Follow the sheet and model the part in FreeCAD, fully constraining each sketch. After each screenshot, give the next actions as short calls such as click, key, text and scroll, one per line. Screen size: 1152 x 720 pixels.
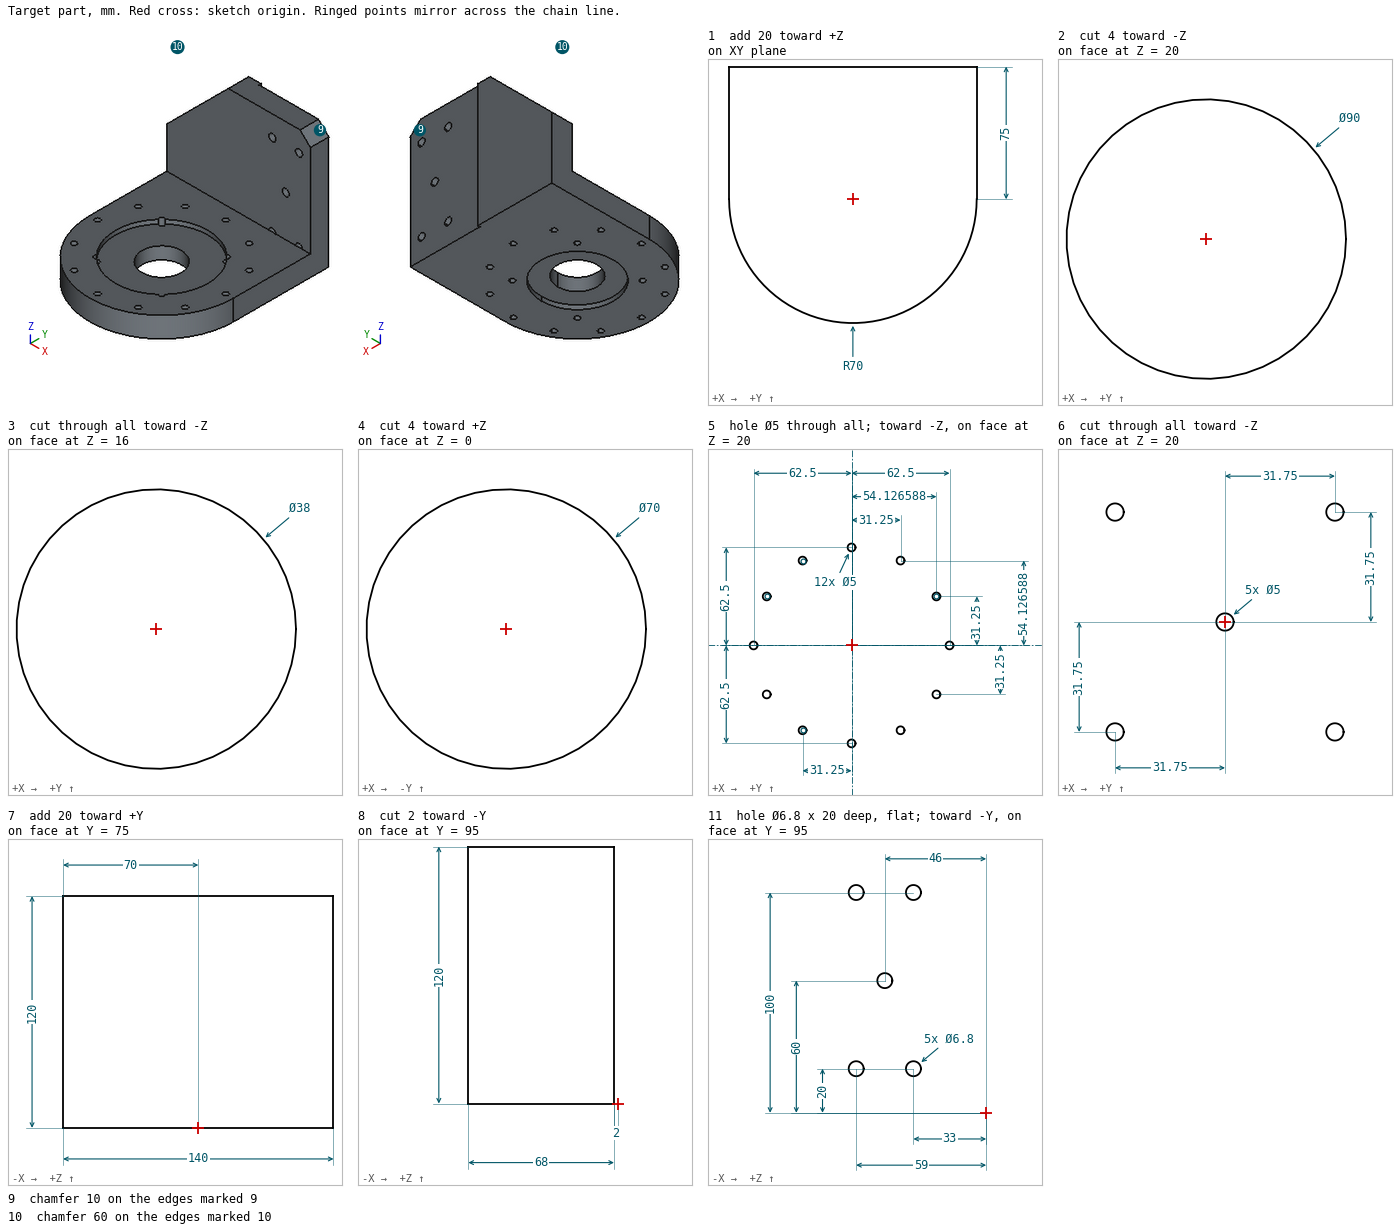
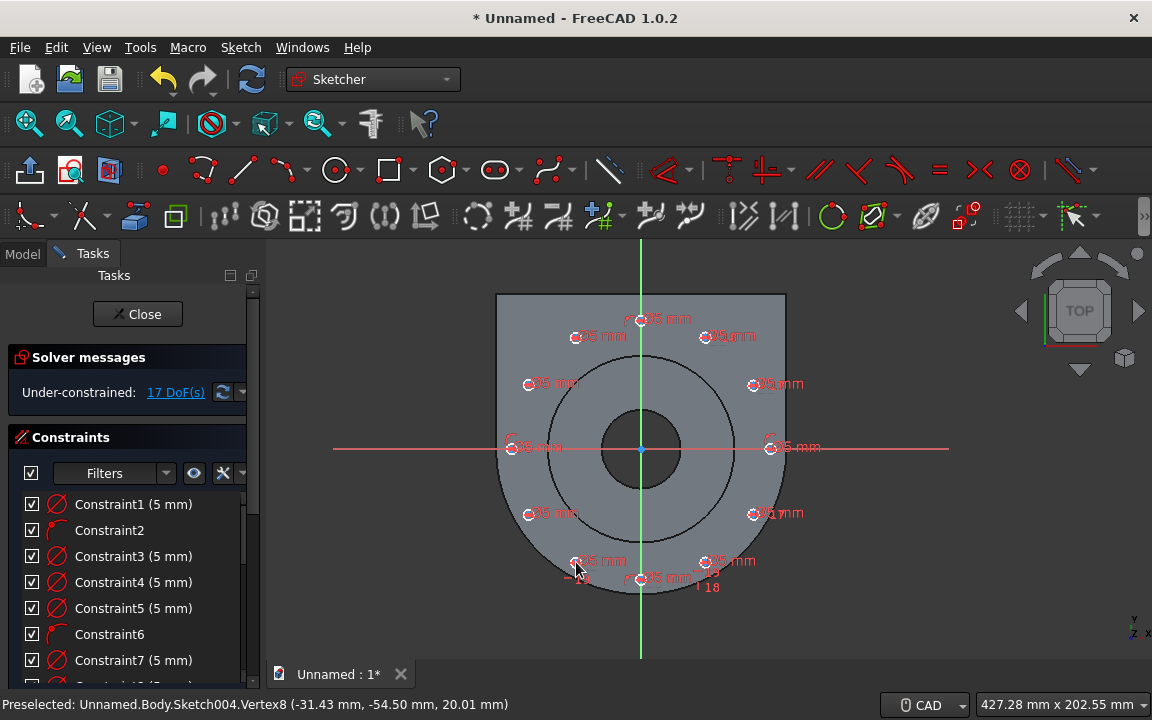
click(754, 515)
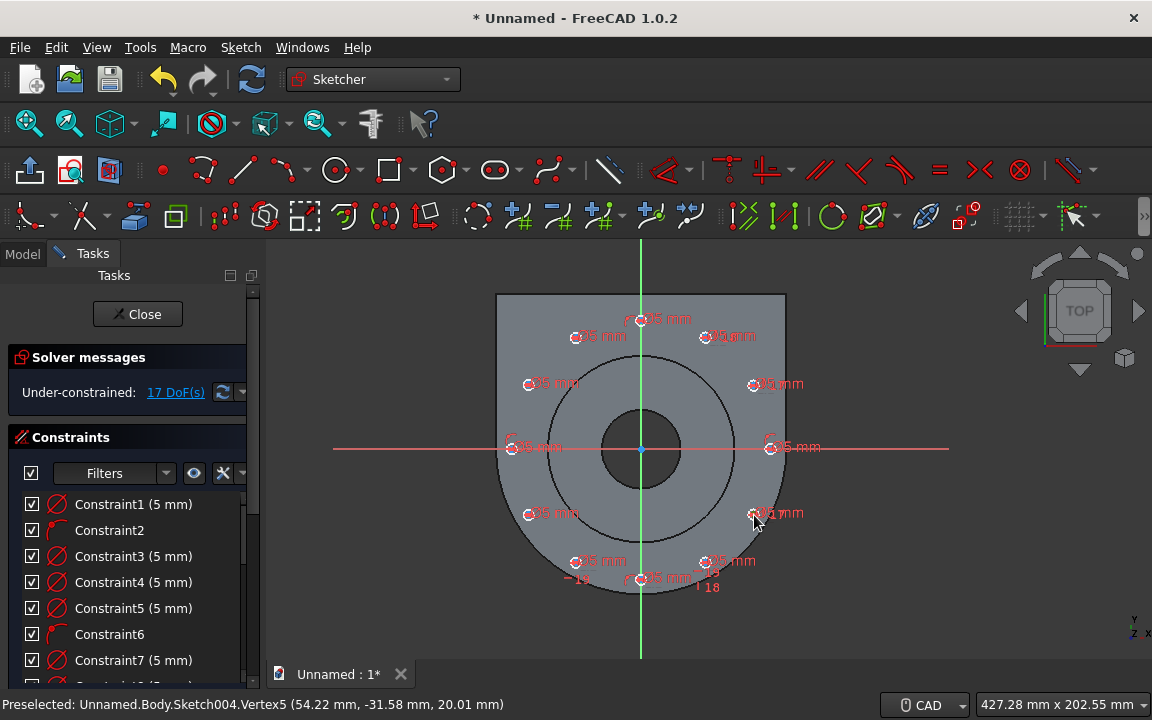
click(529, 515)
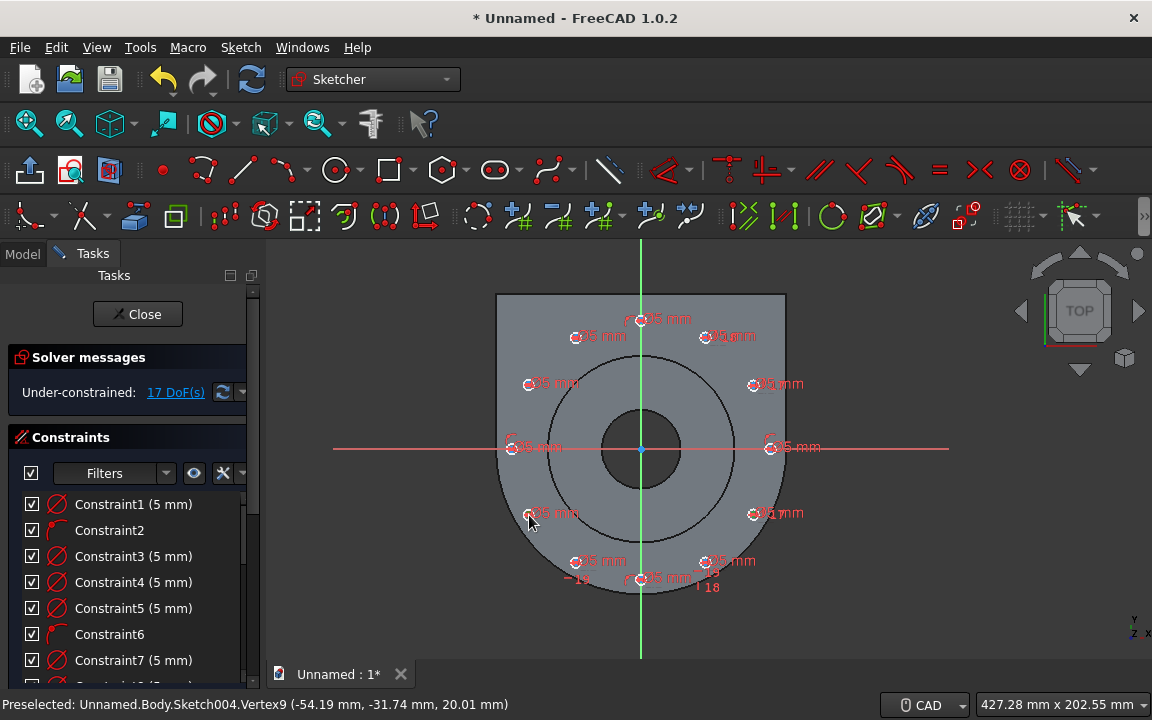
key(h)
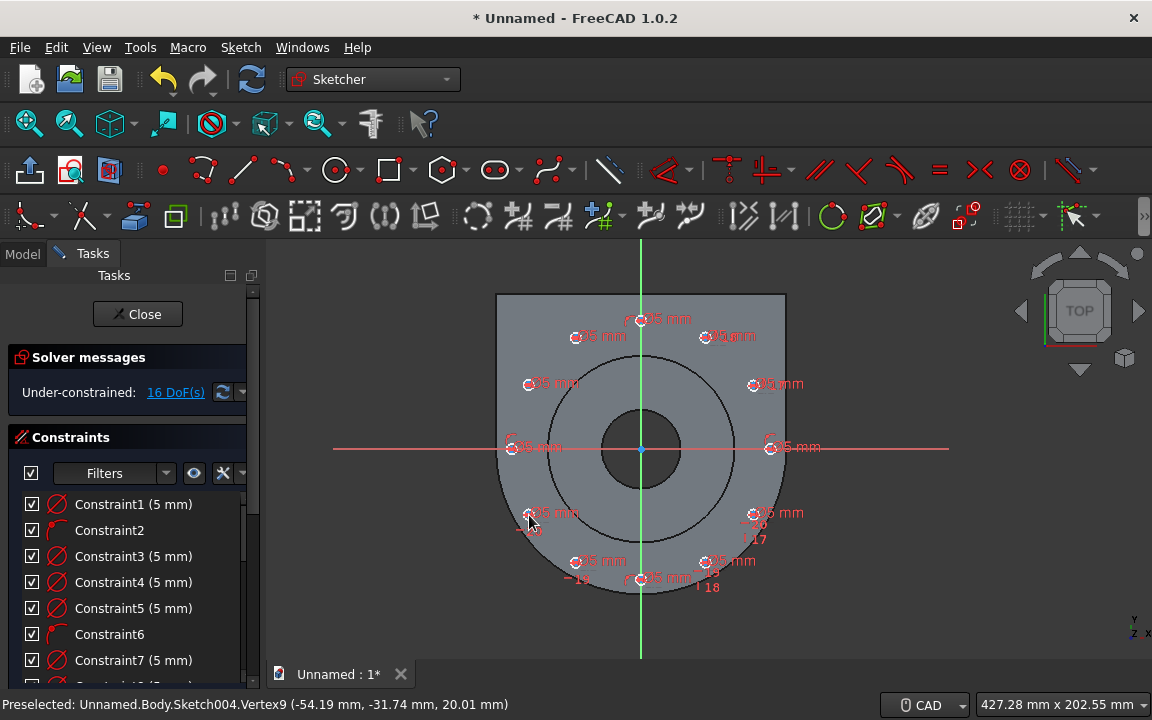
click(529, 515)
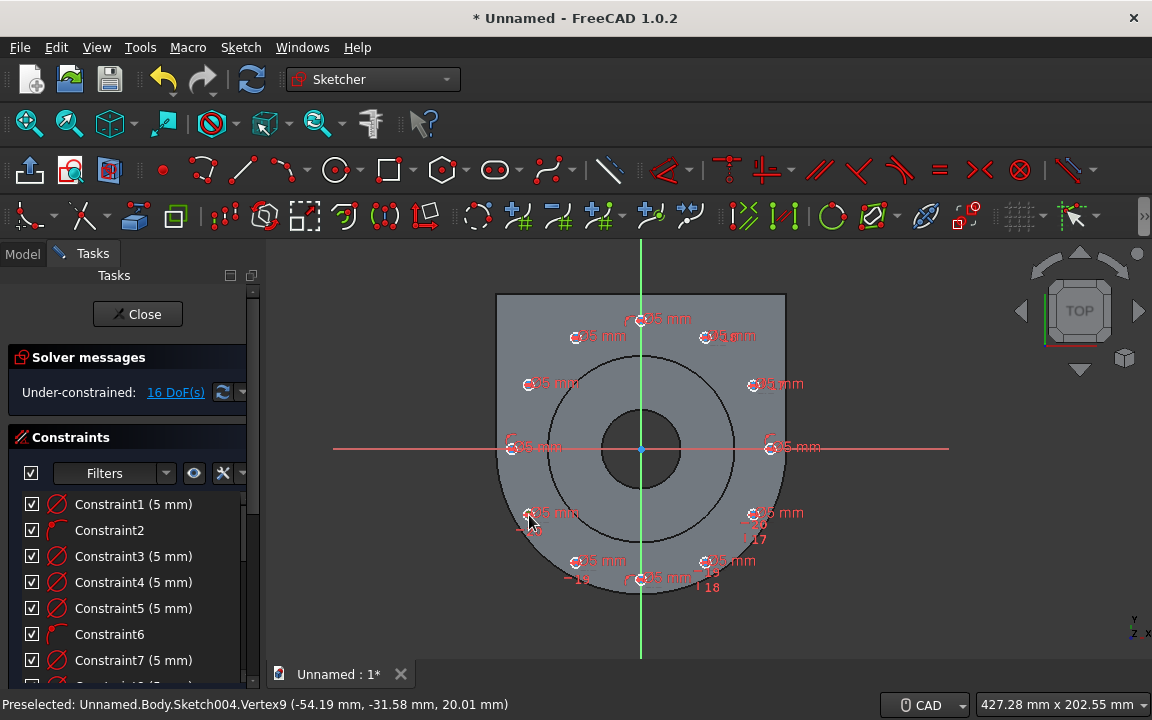
click(529, 385)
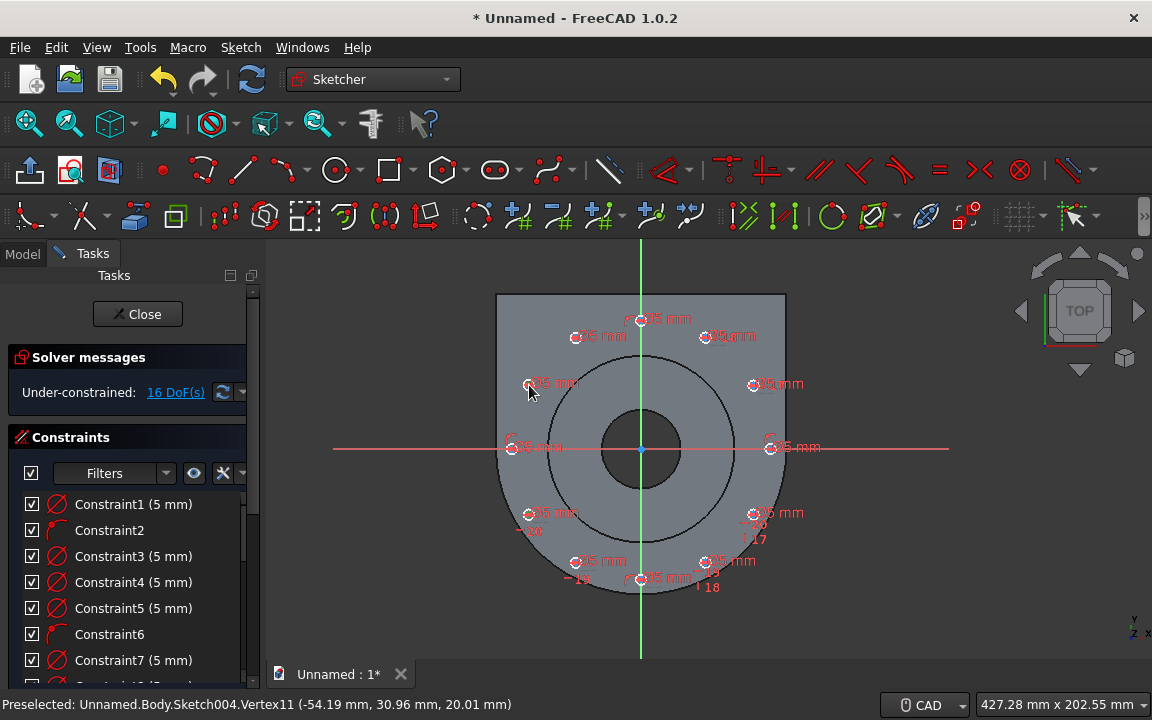
key(v)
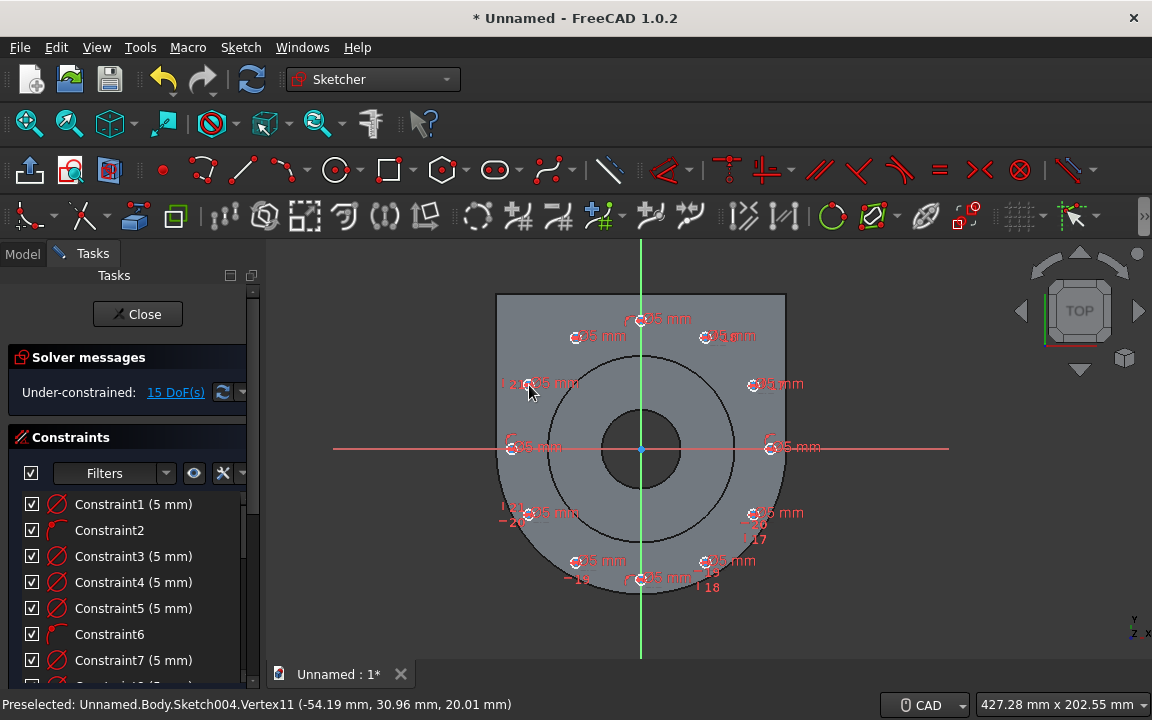
click(706, 338)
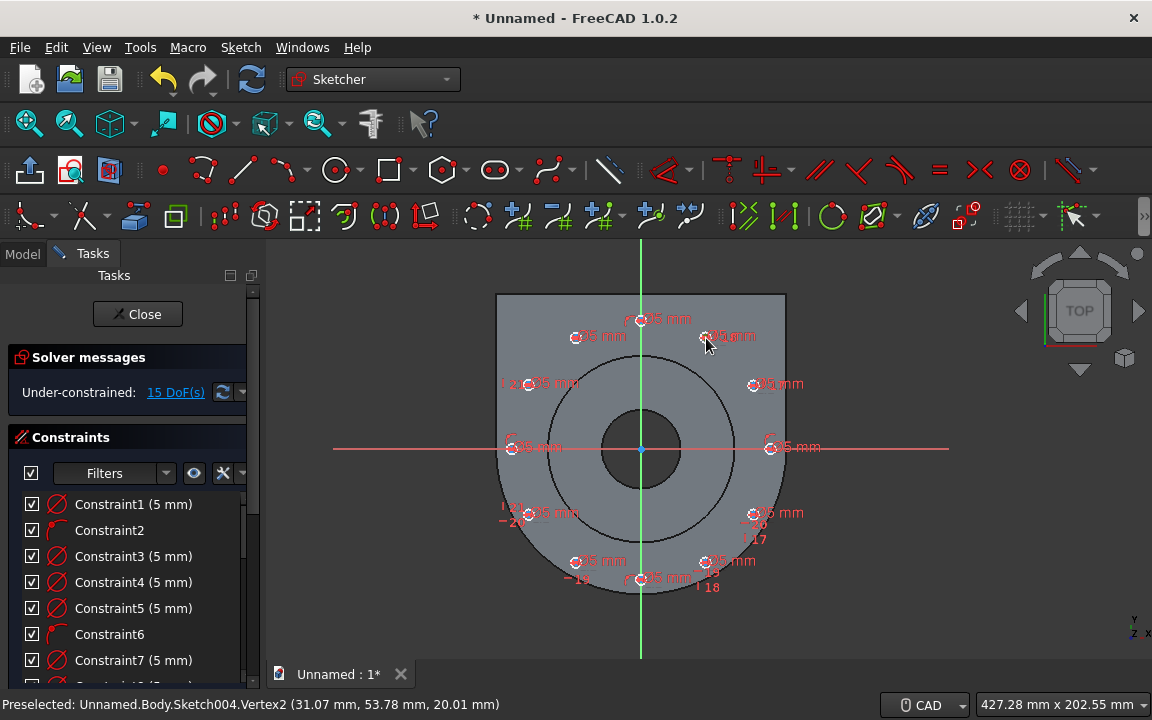
click(576, 338)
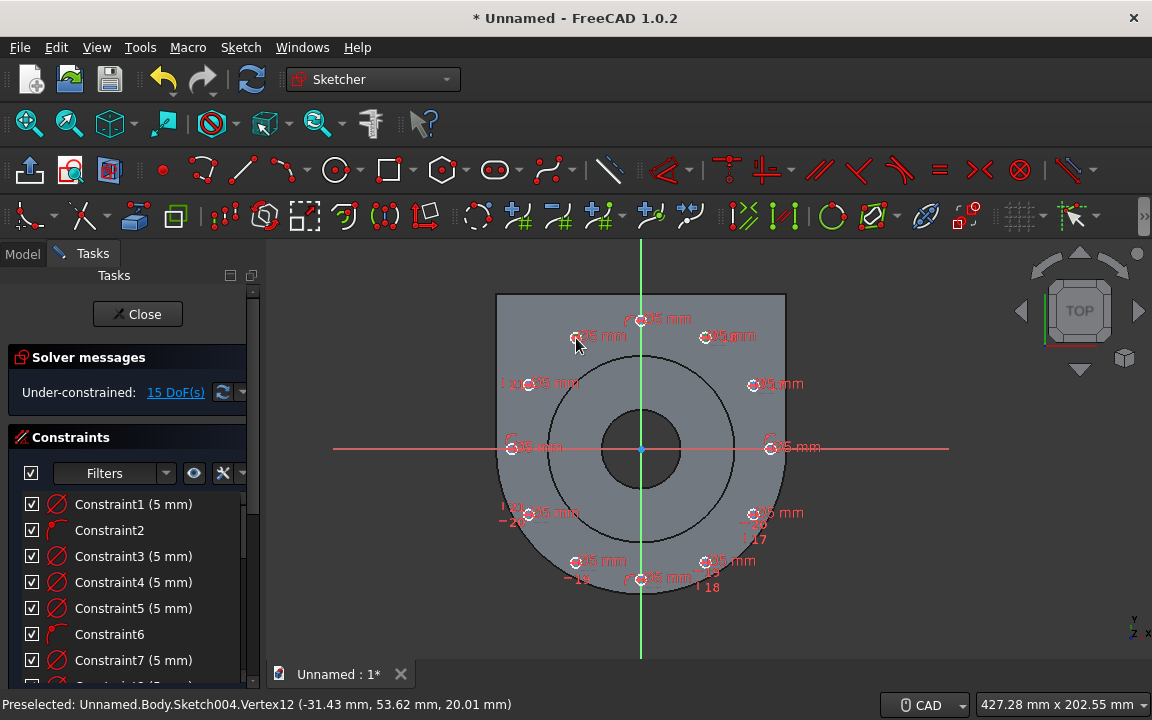
key(h)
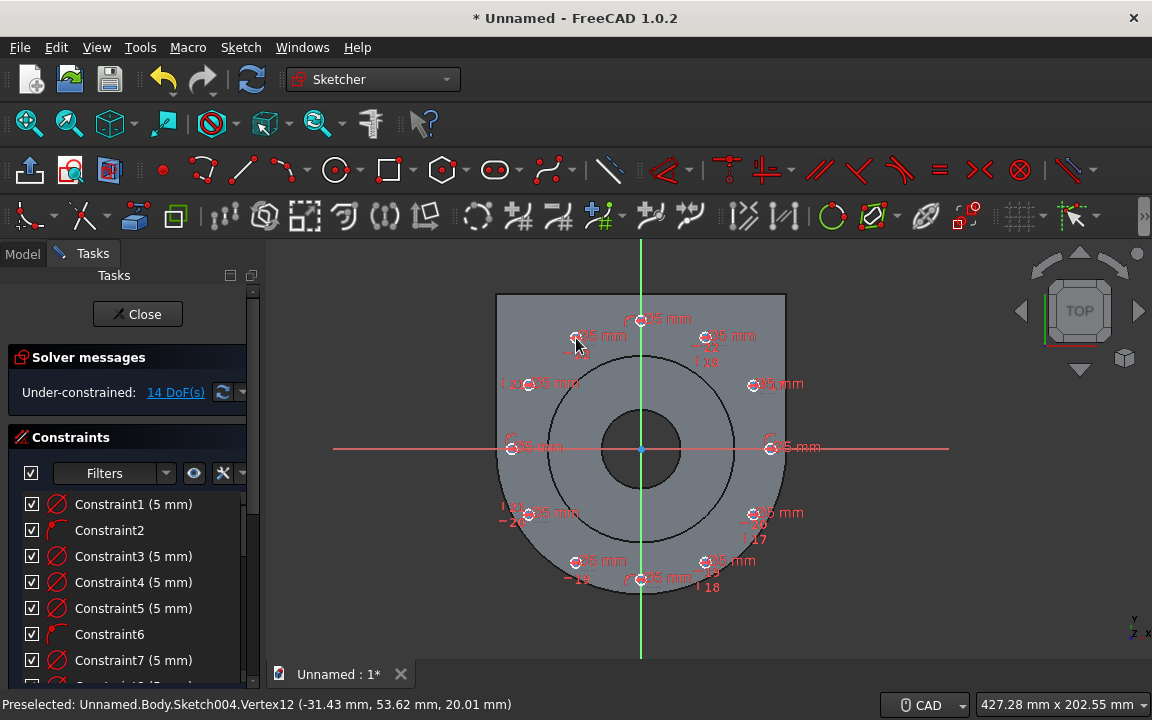
click(754, 386)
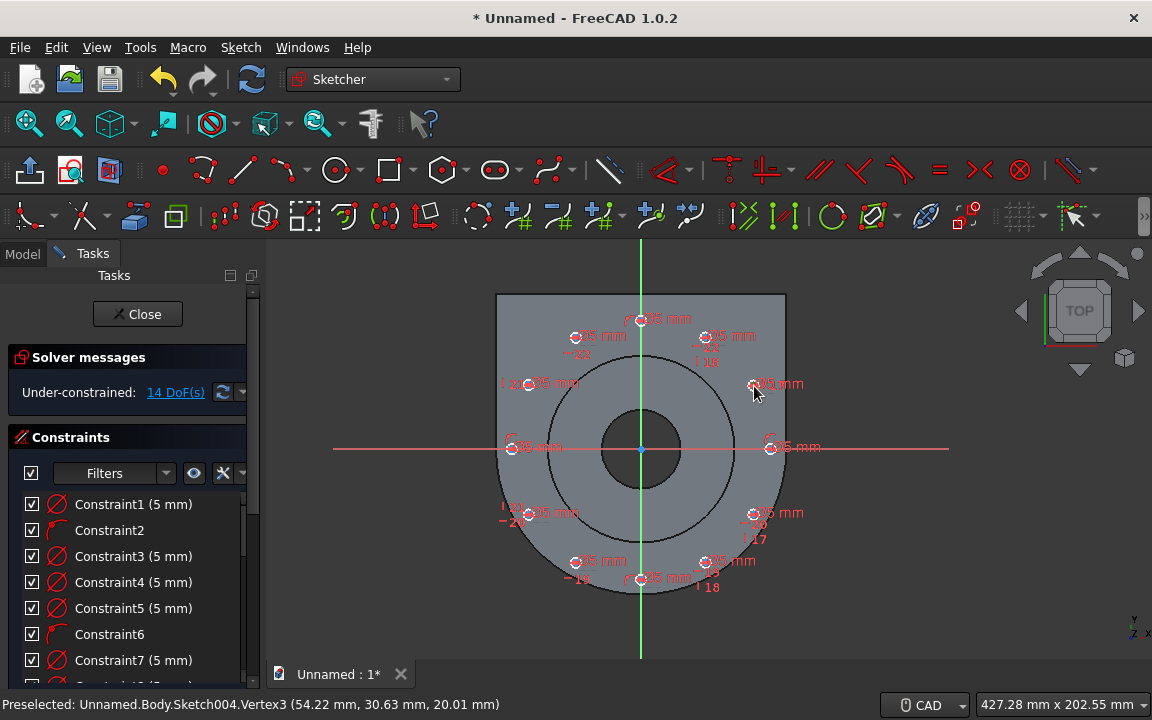
click(529, 385)